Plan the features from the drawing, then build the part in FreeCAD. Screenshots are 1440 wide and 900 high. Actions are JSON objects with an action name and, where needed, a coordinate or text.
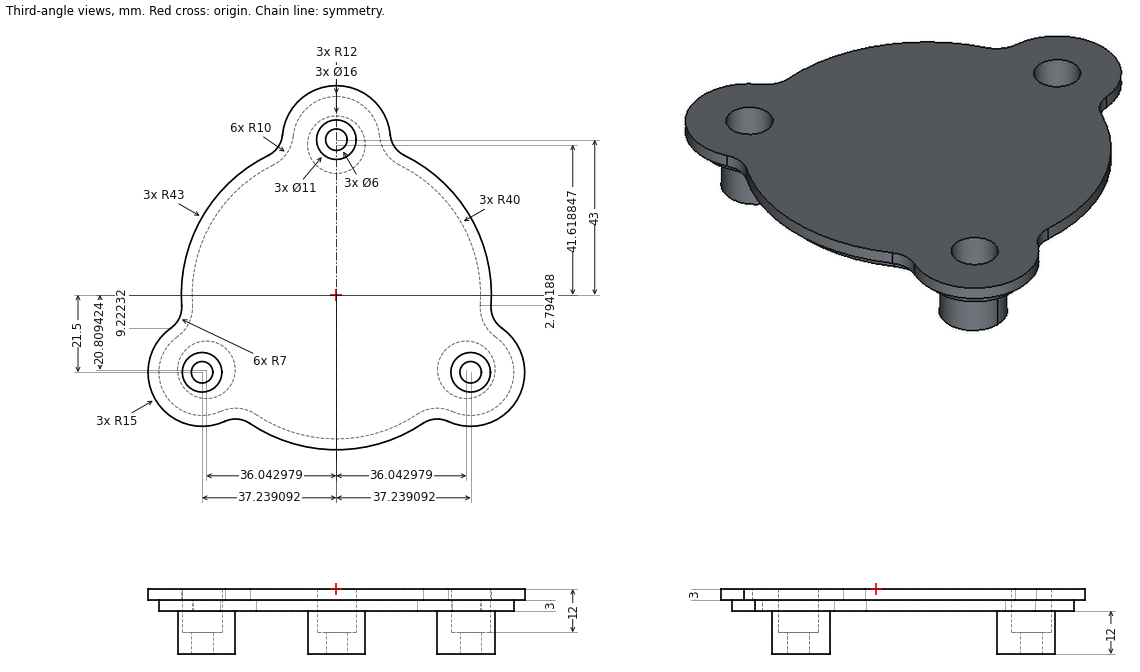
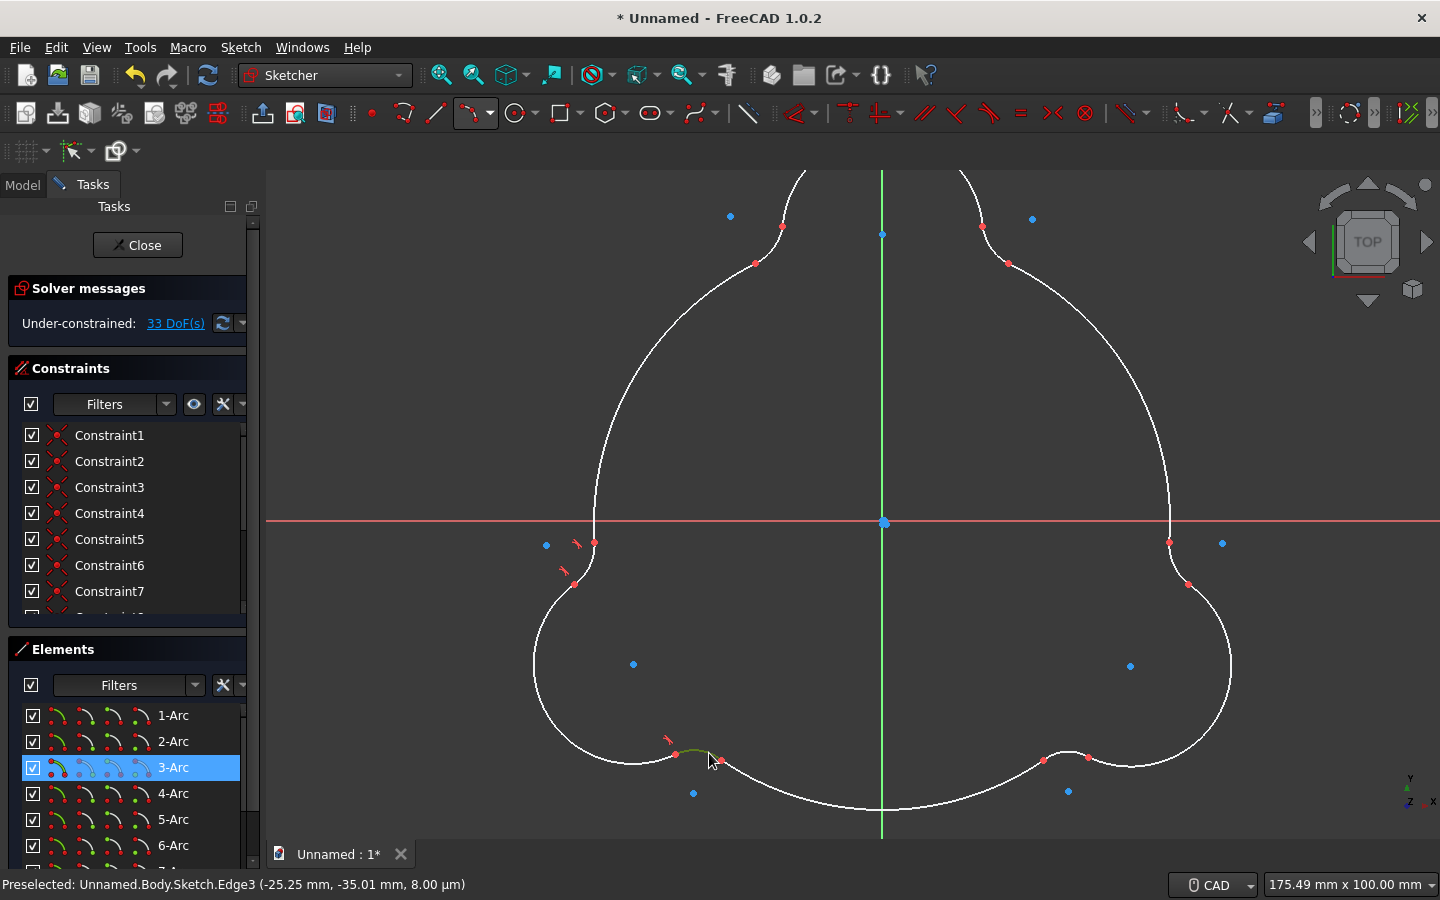
{"action": "left_click", "coordinate": [815, 802]}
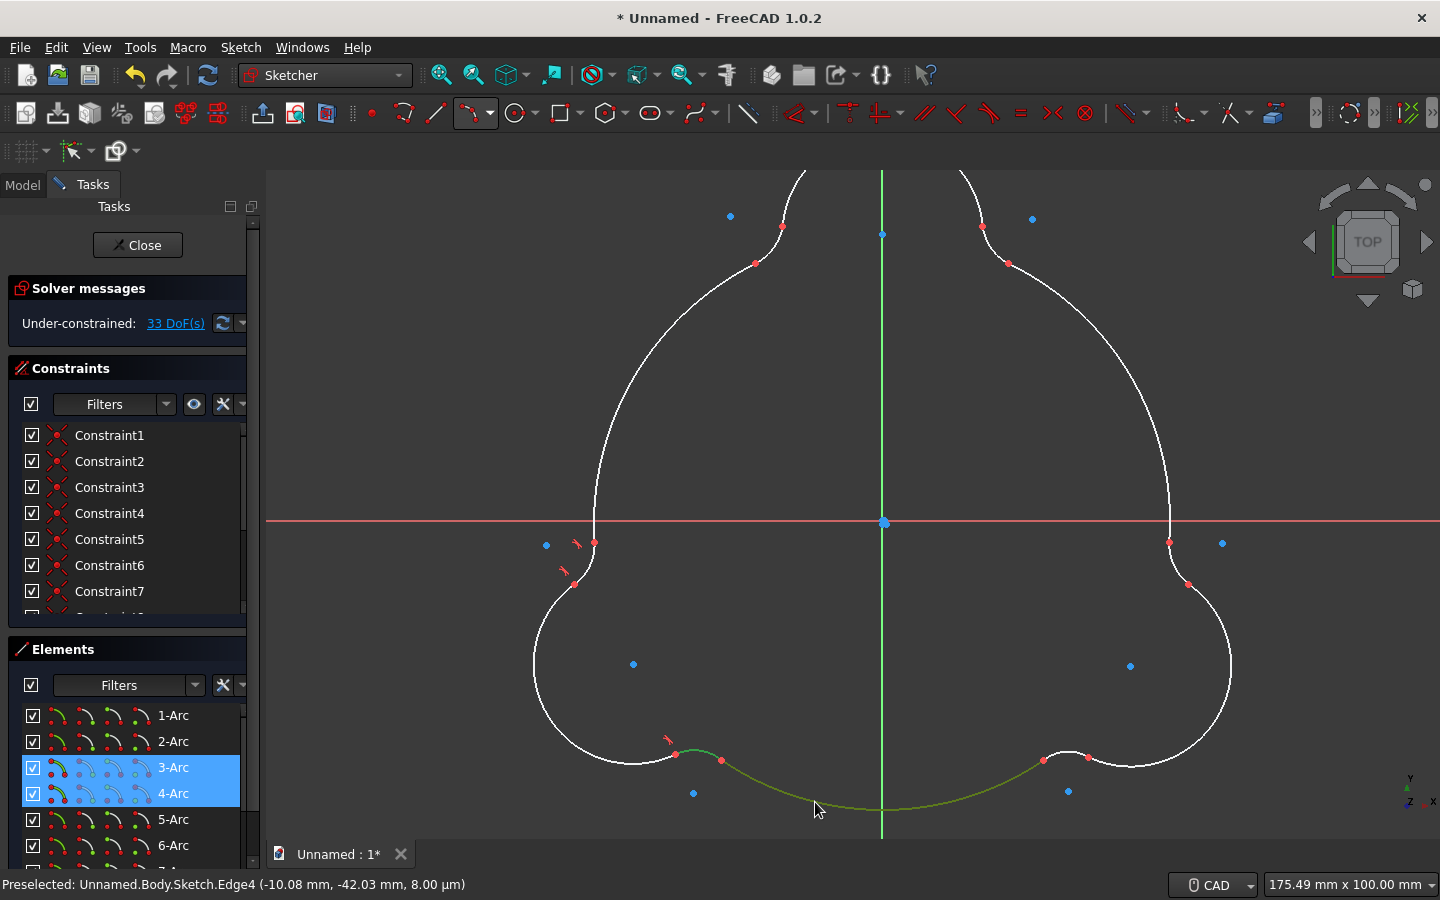
{"action": "left_click", "coordinate": [990, 114]}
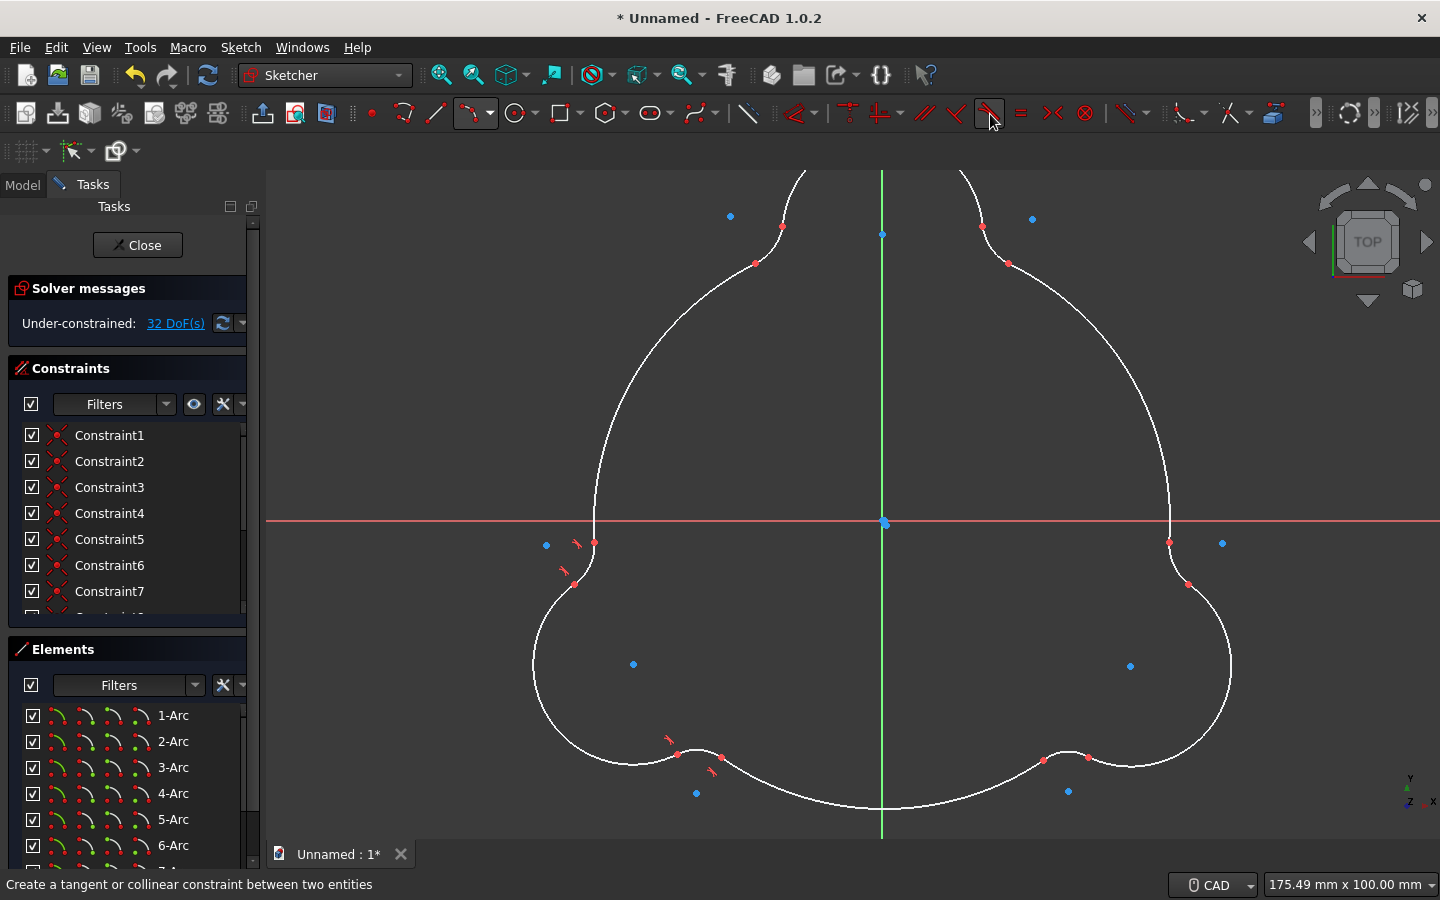
{"action": "left_click", "coordinate": [815, 800]}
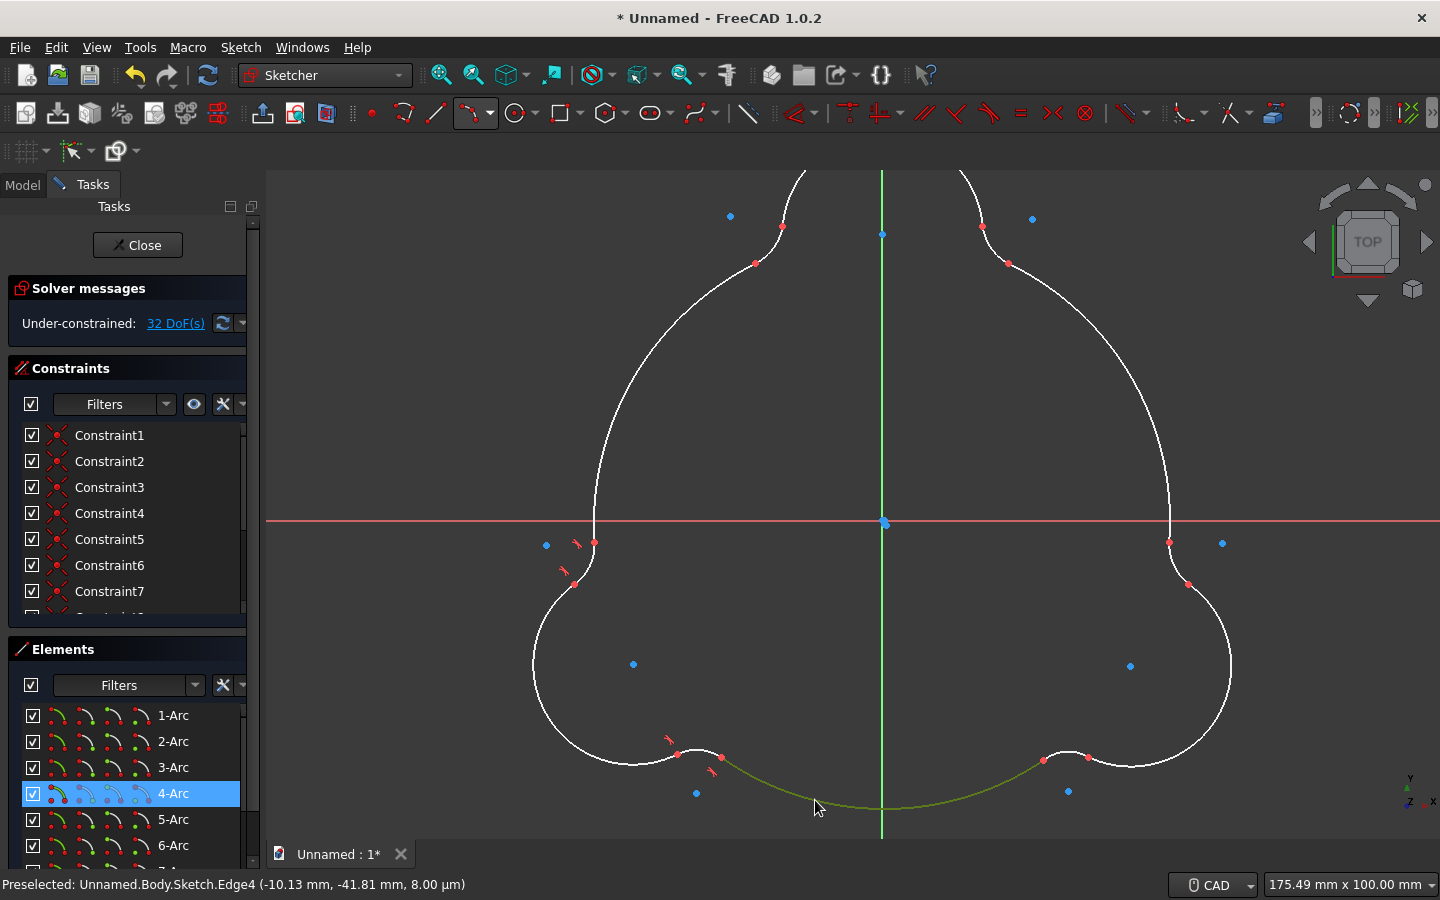
{"action": "left_click", "coordinate": [1075, 752]}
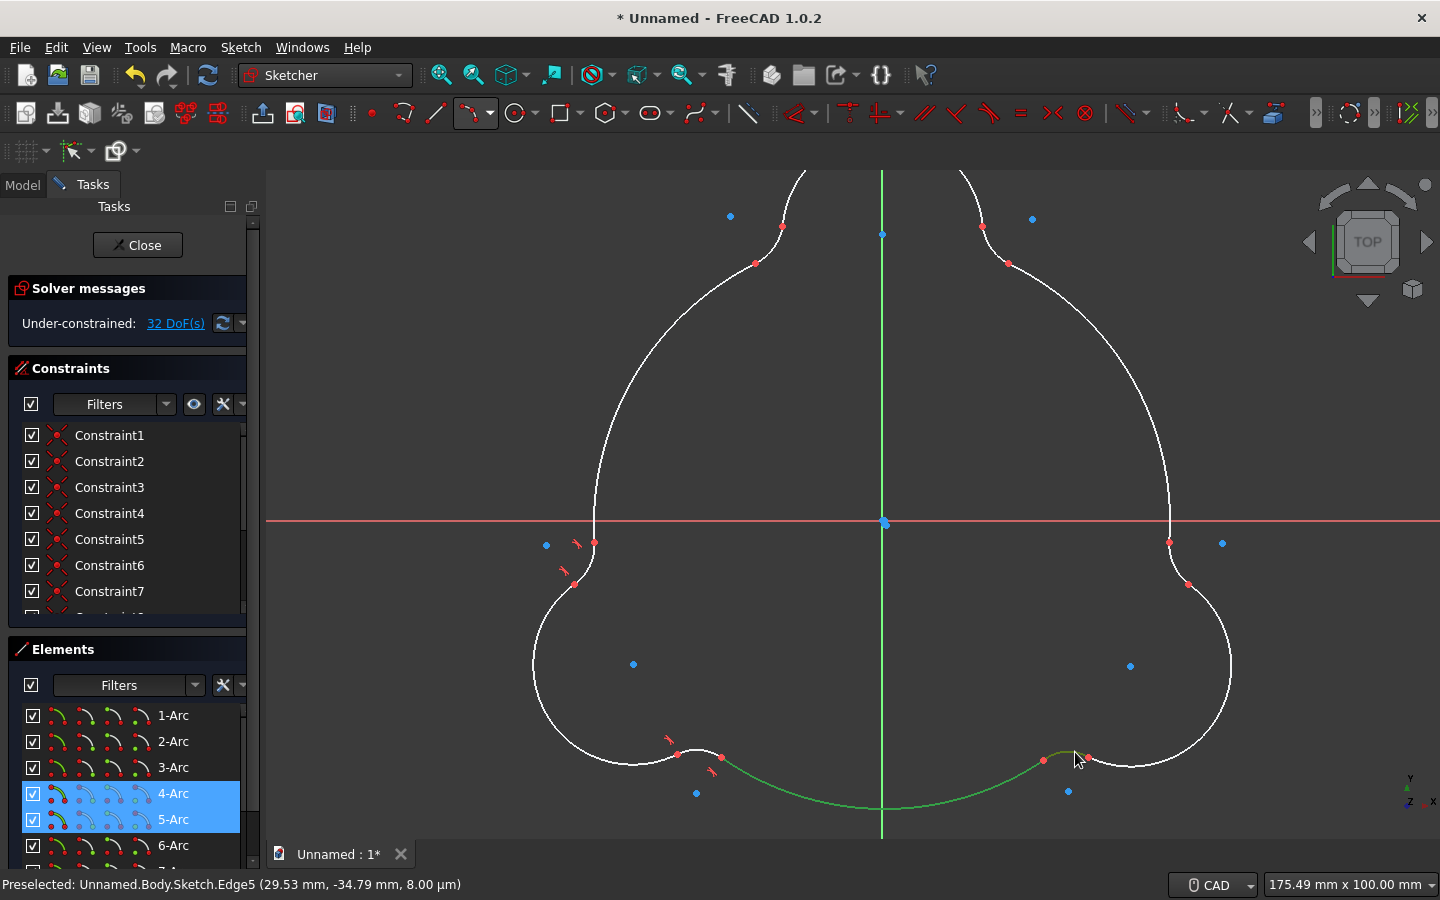
{"action": "left_click", "coordinate": [990, 114]}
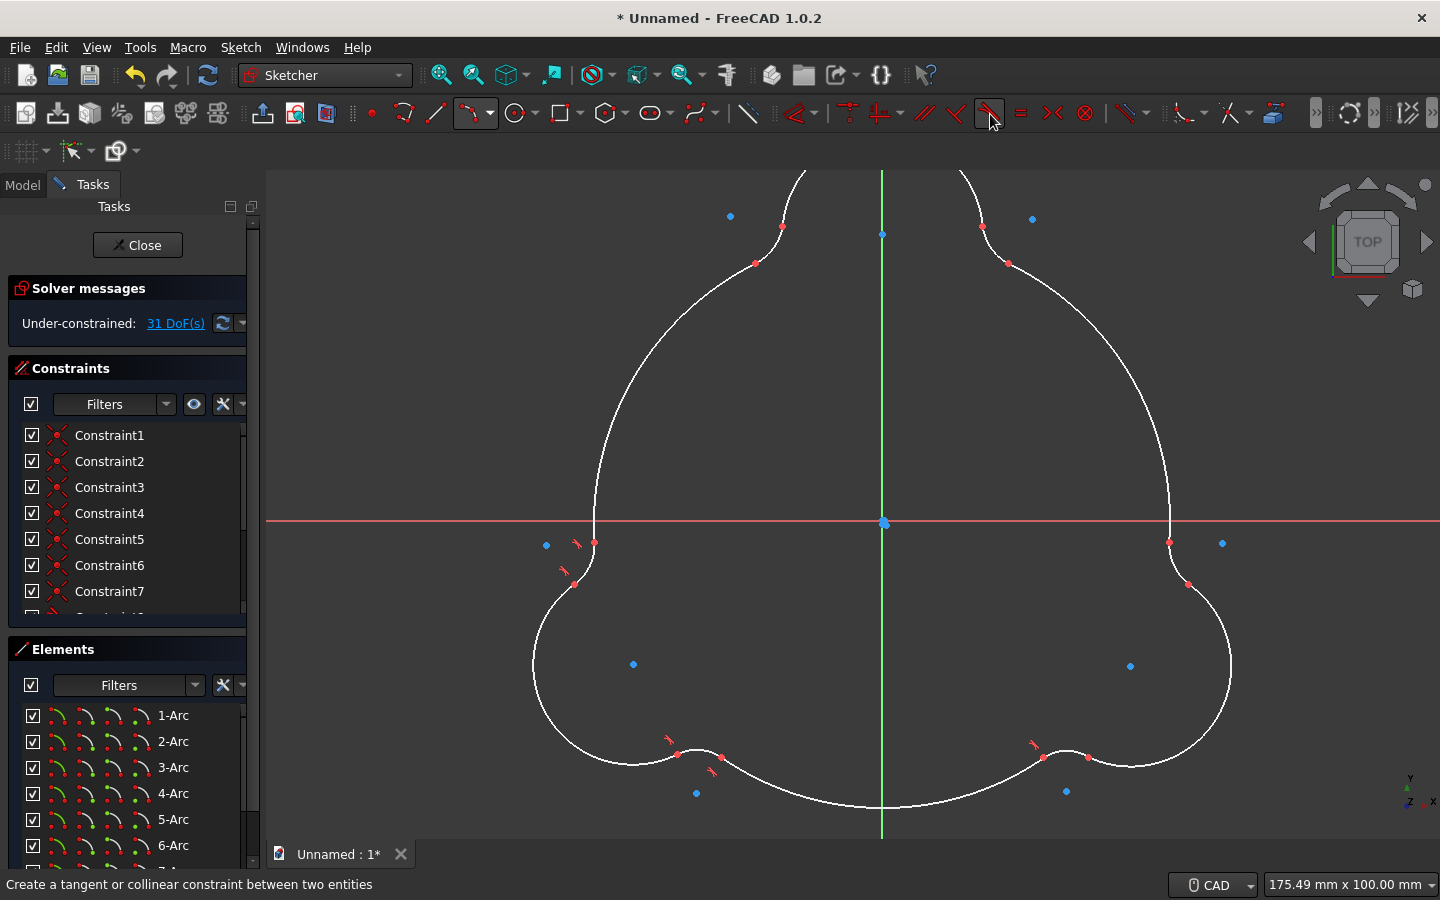
{"action": "left_click", "coordinate": [1076, 752]}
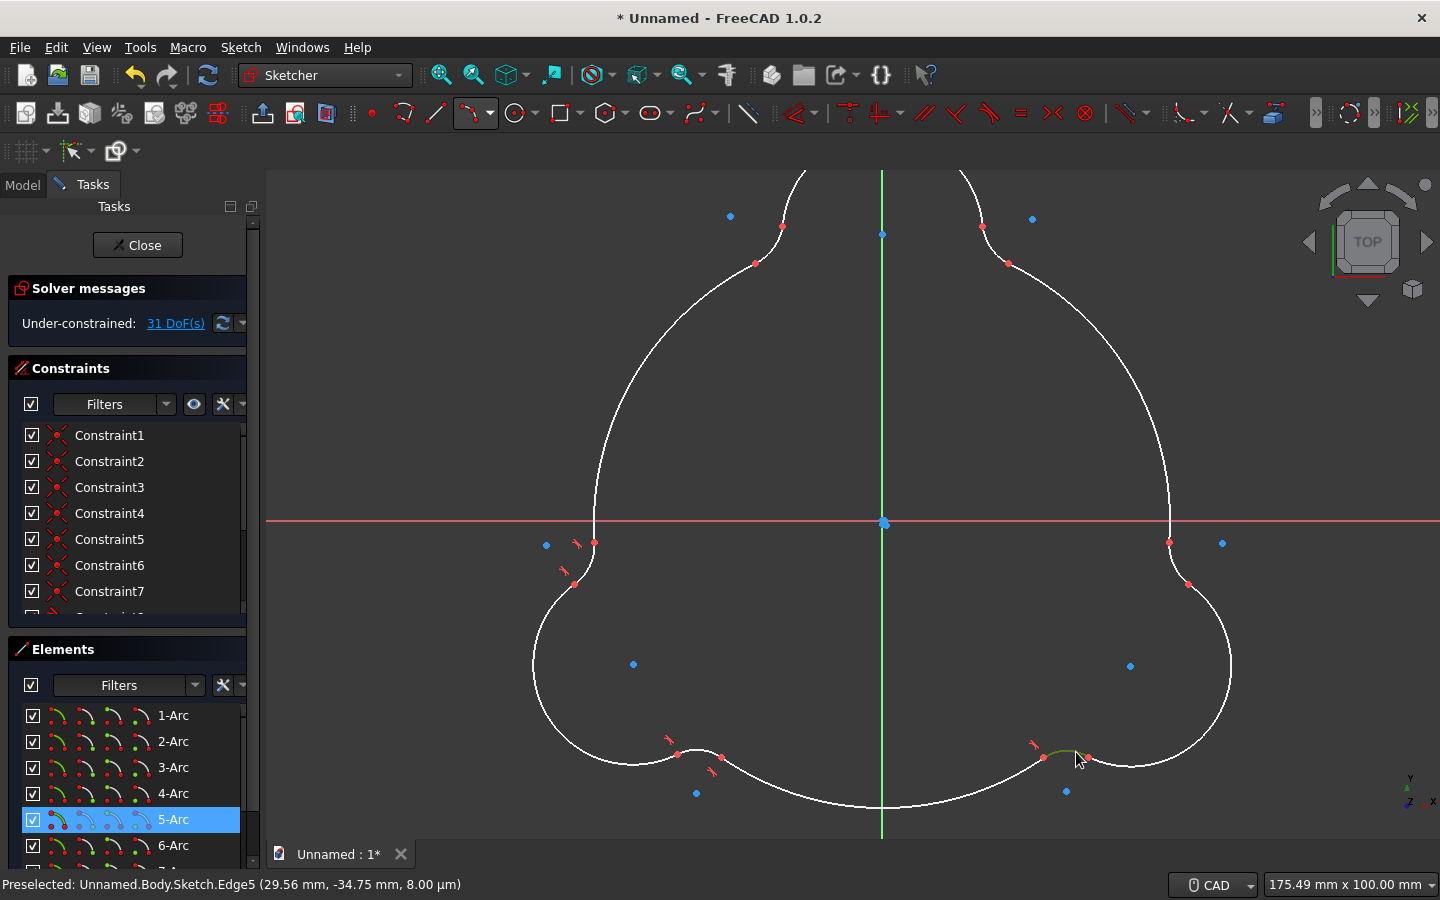
{"action": "left_click", "coordinate": [1175, 756]}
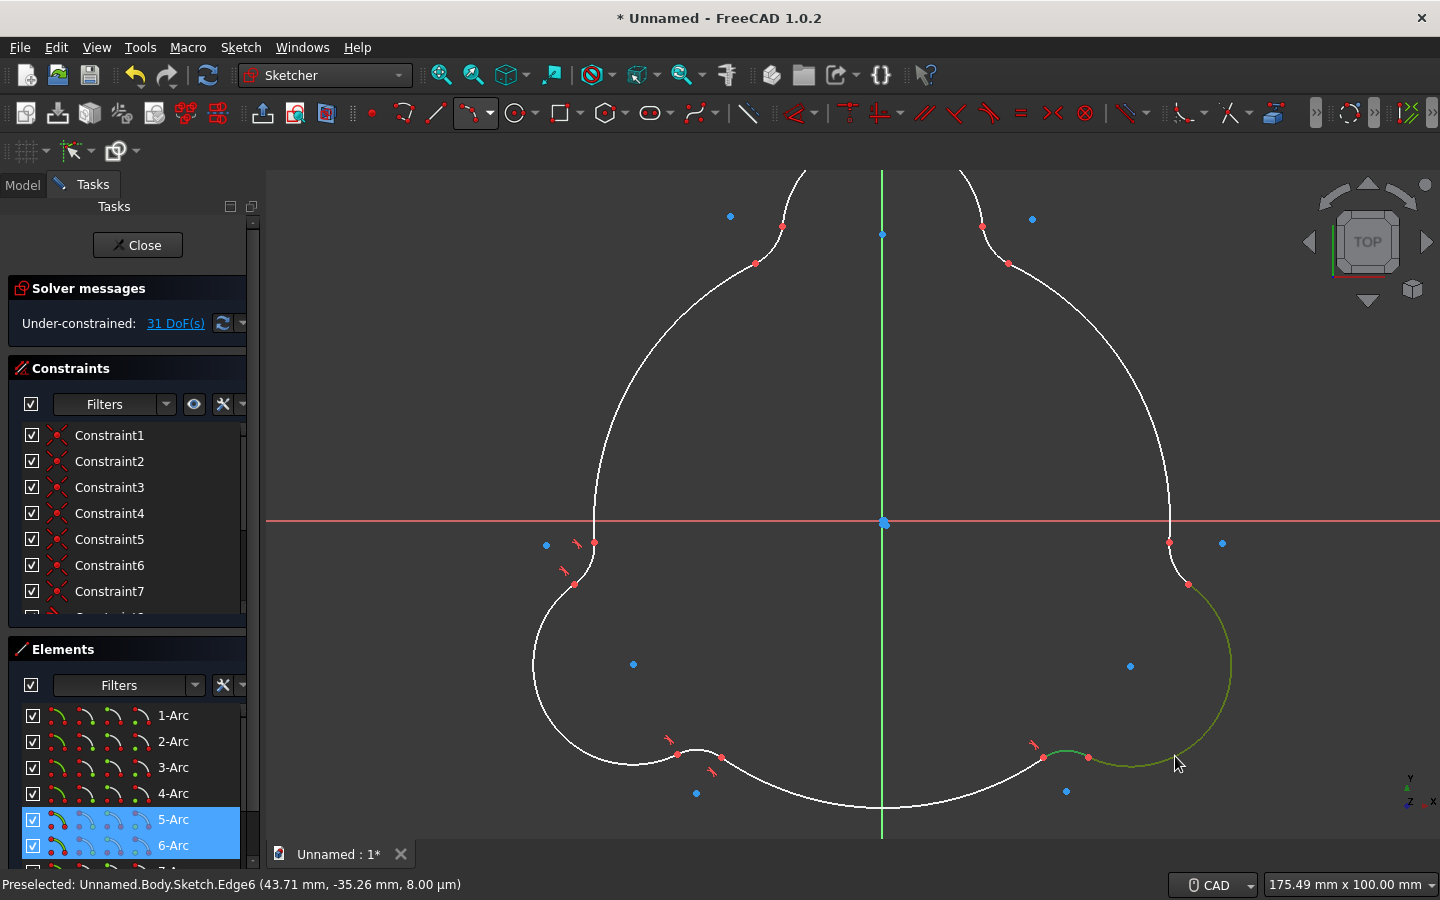
{"action": "left_click", "coordinate": [990, 114]}